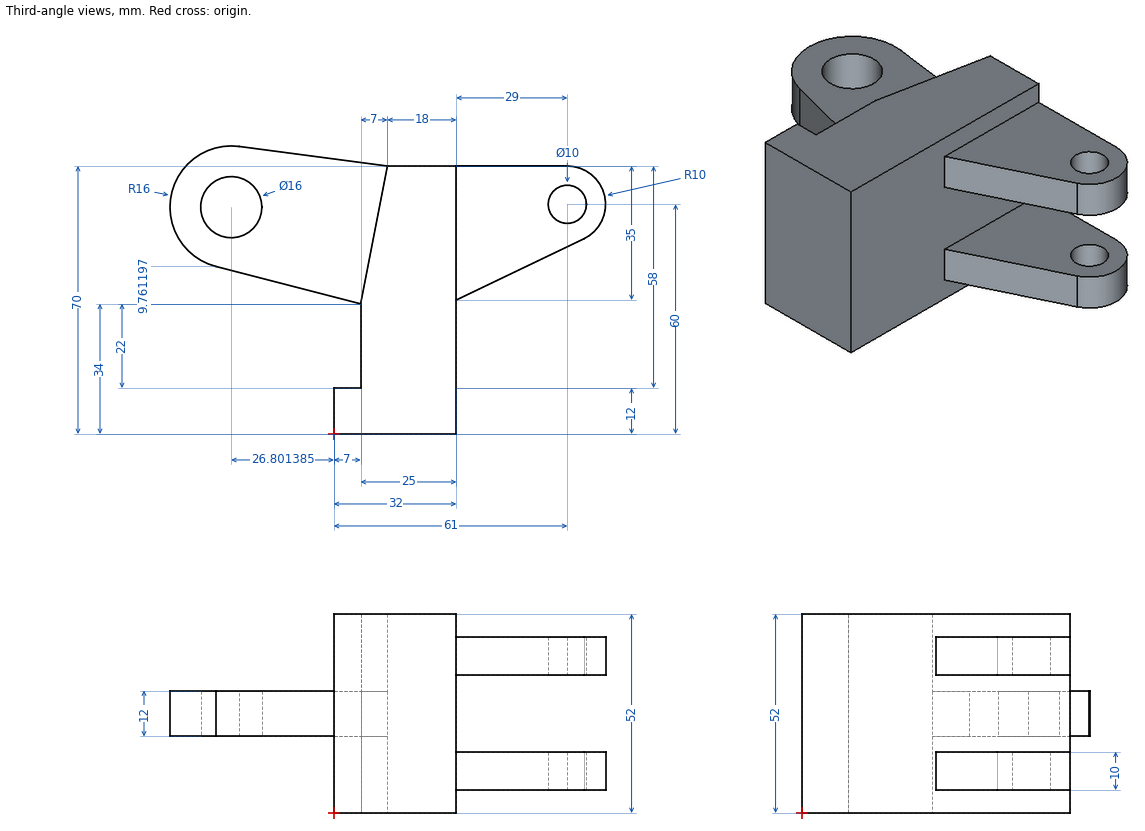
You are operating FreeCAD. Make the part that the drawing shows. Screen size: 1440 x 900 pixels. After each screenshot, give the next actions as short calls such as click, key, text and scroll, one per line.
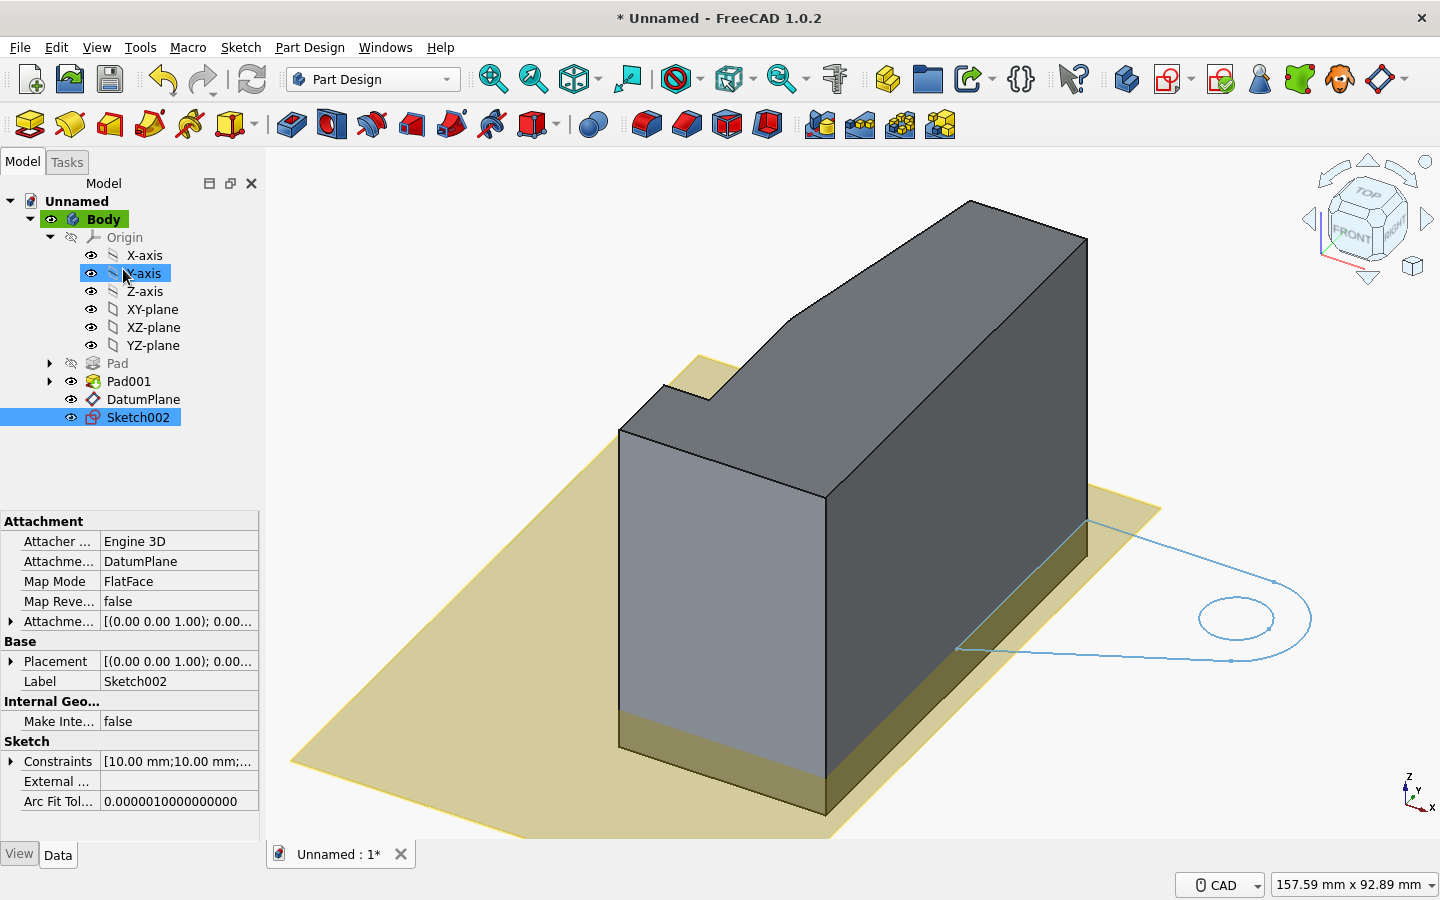
click(30, 124)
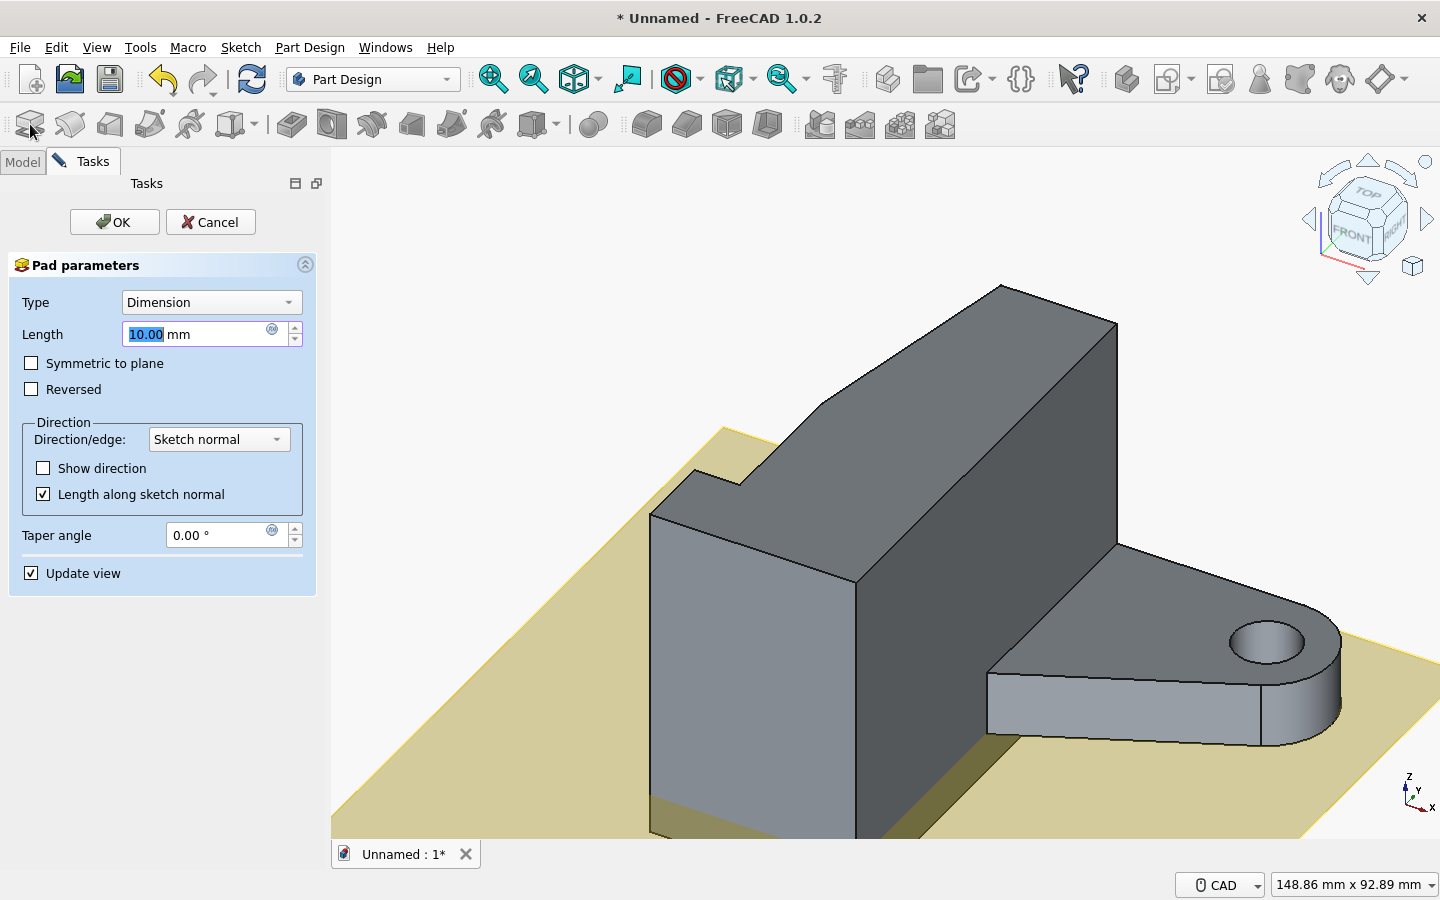
text(10)
key(Tab)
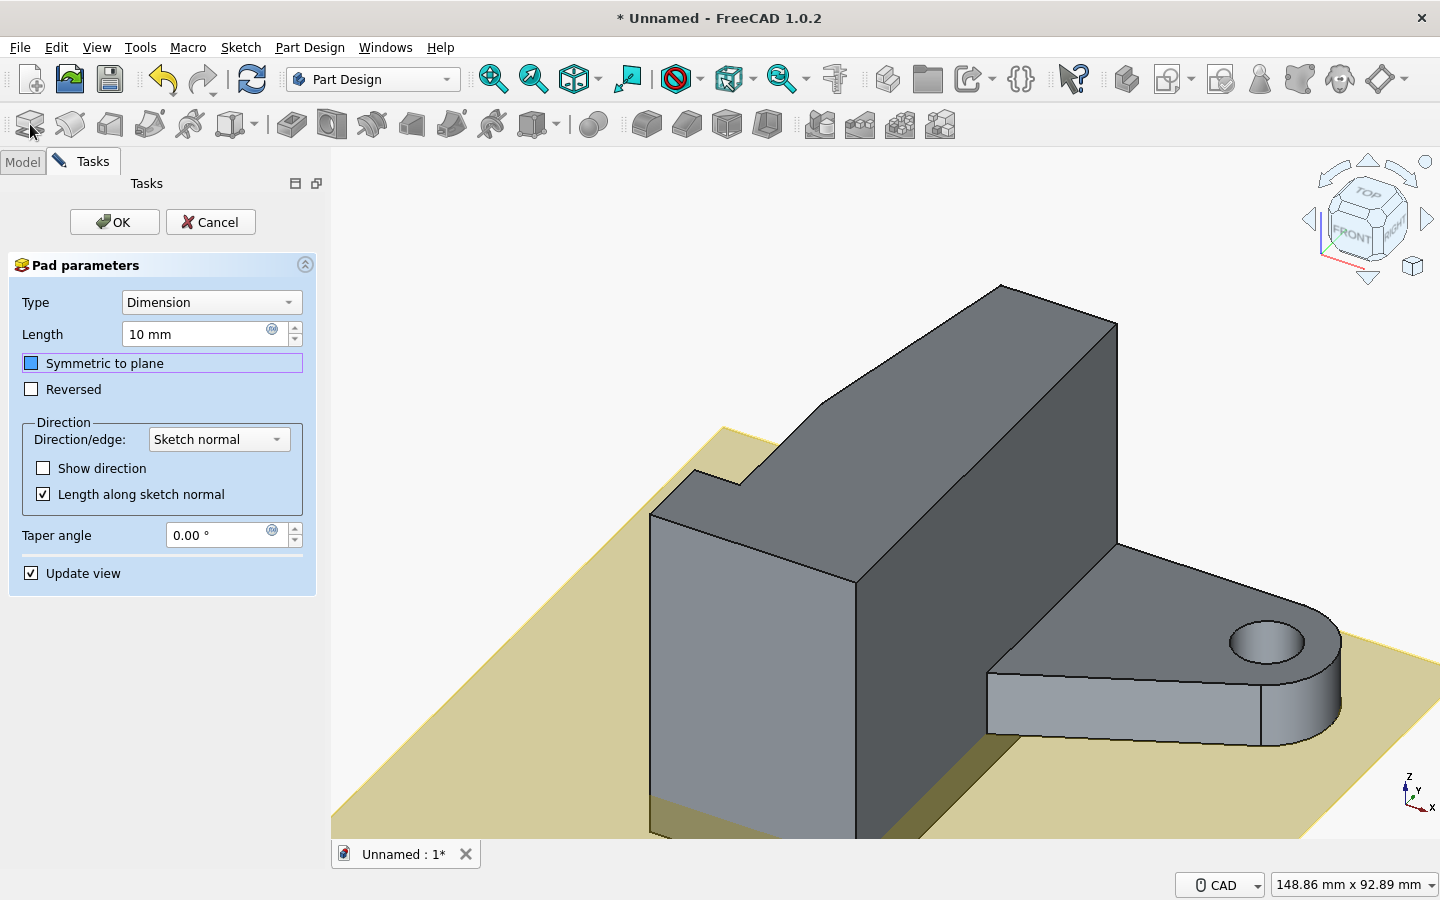
click(115, 222)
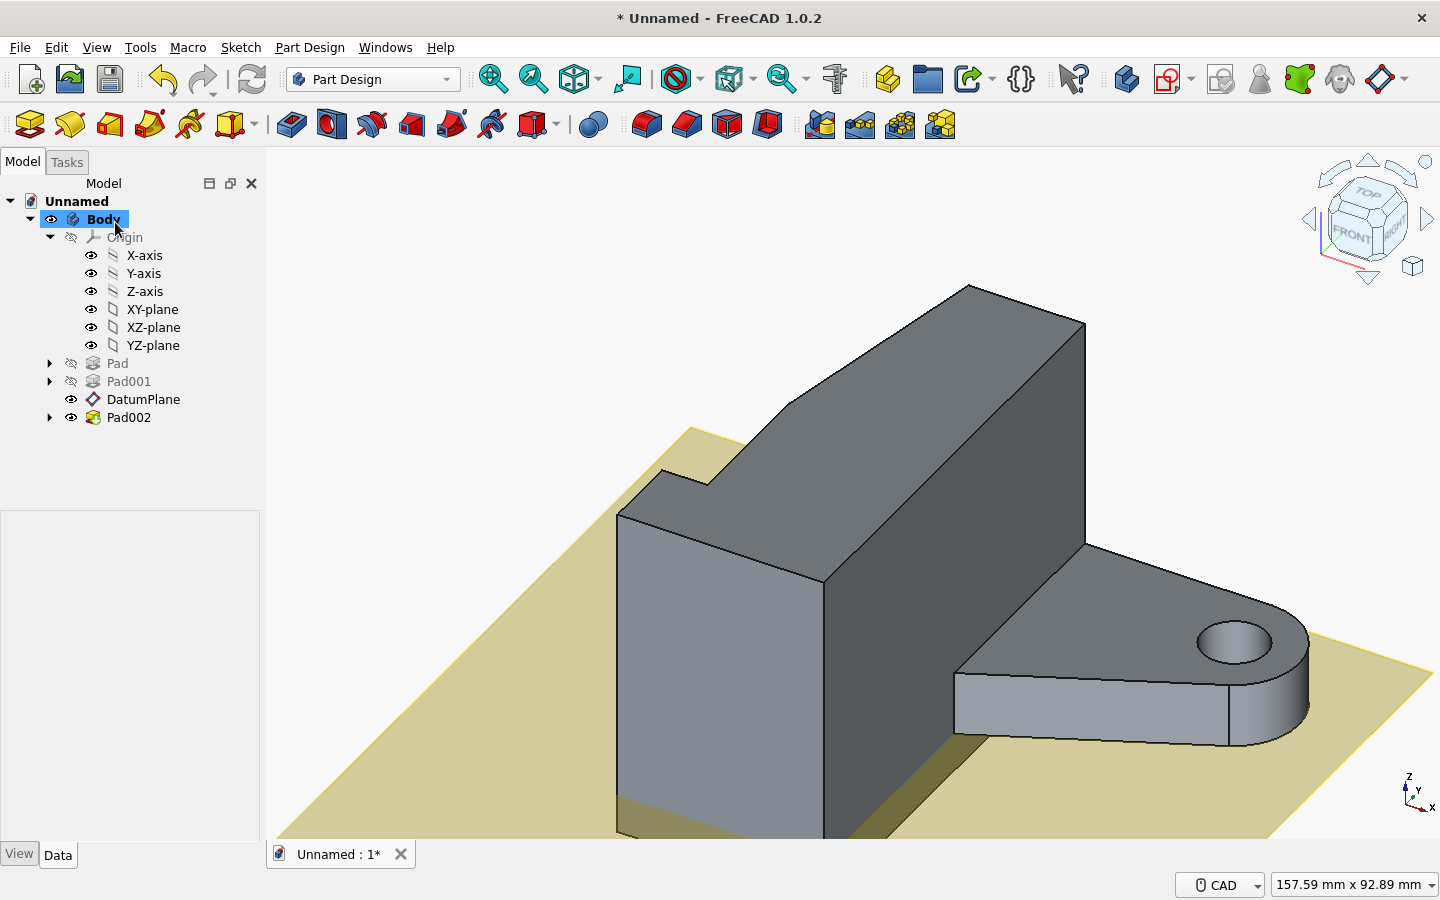
click(116, 399)
key(space)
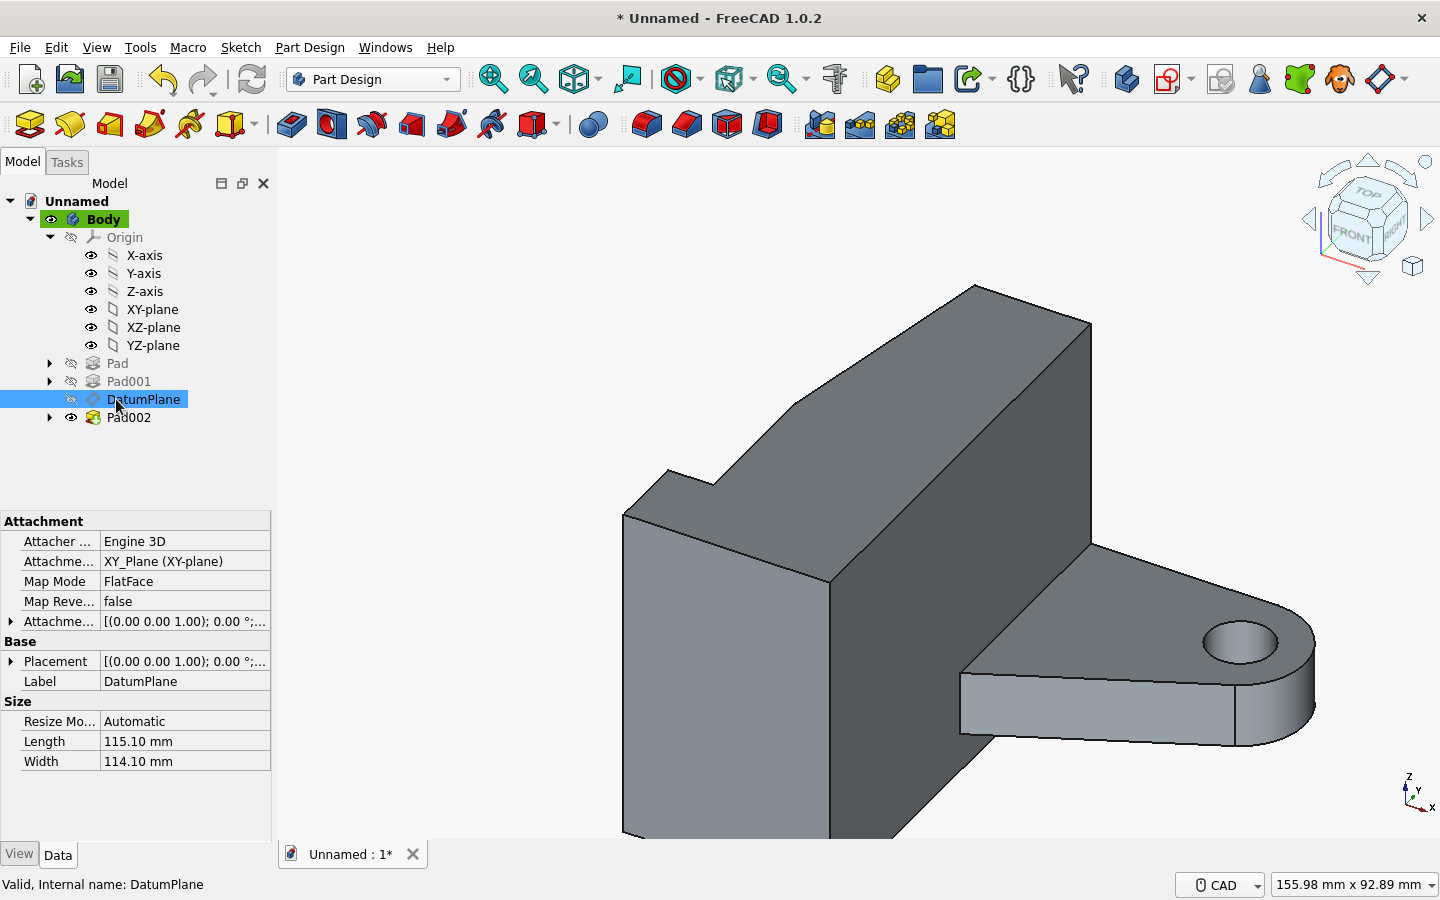
click(494, 80)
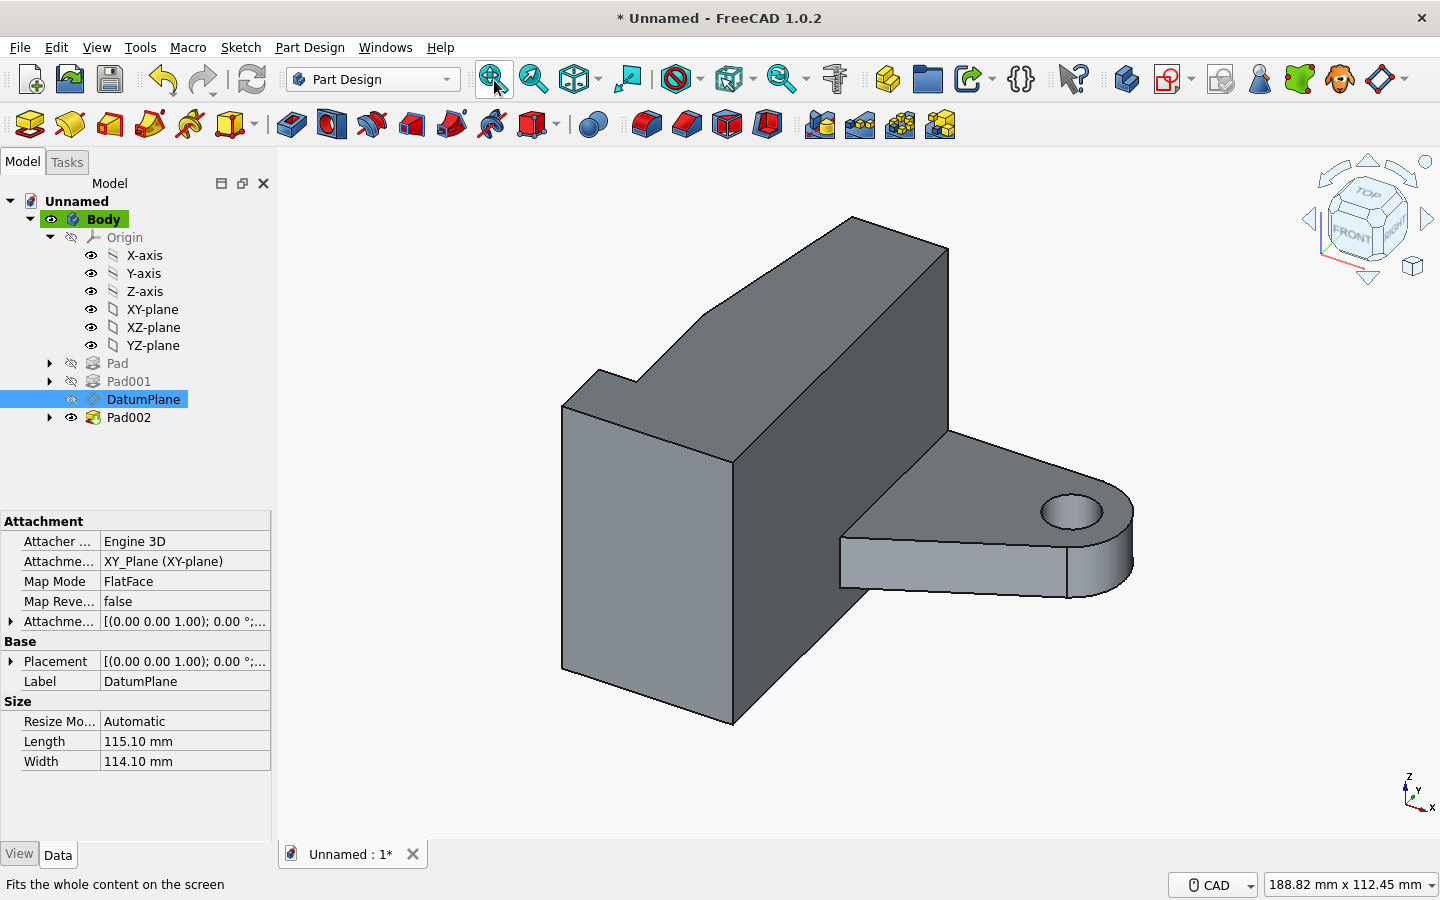
click(136, 309)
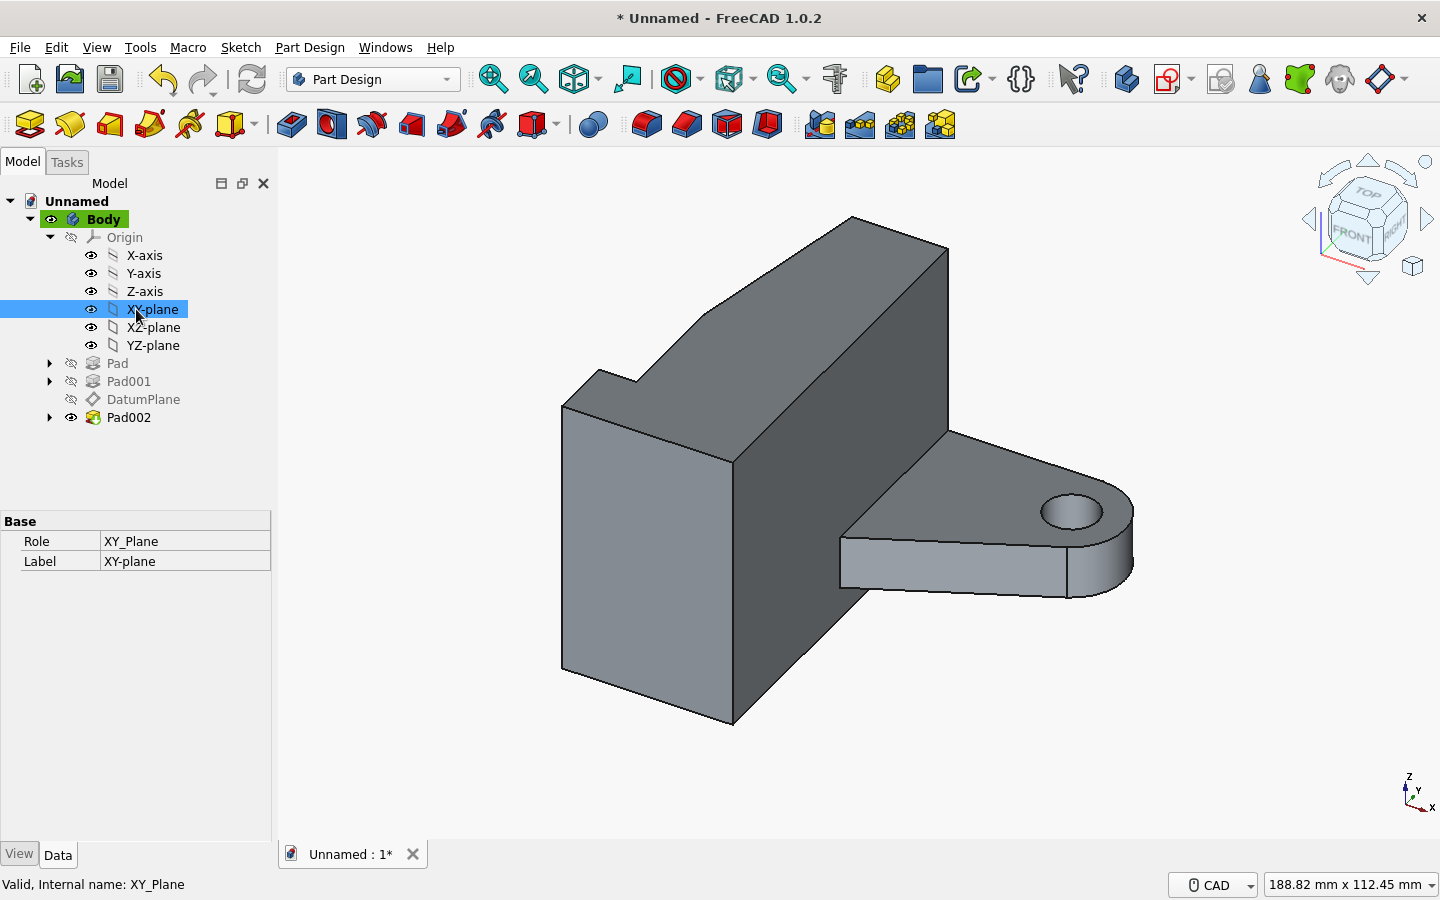
click(1380, 80)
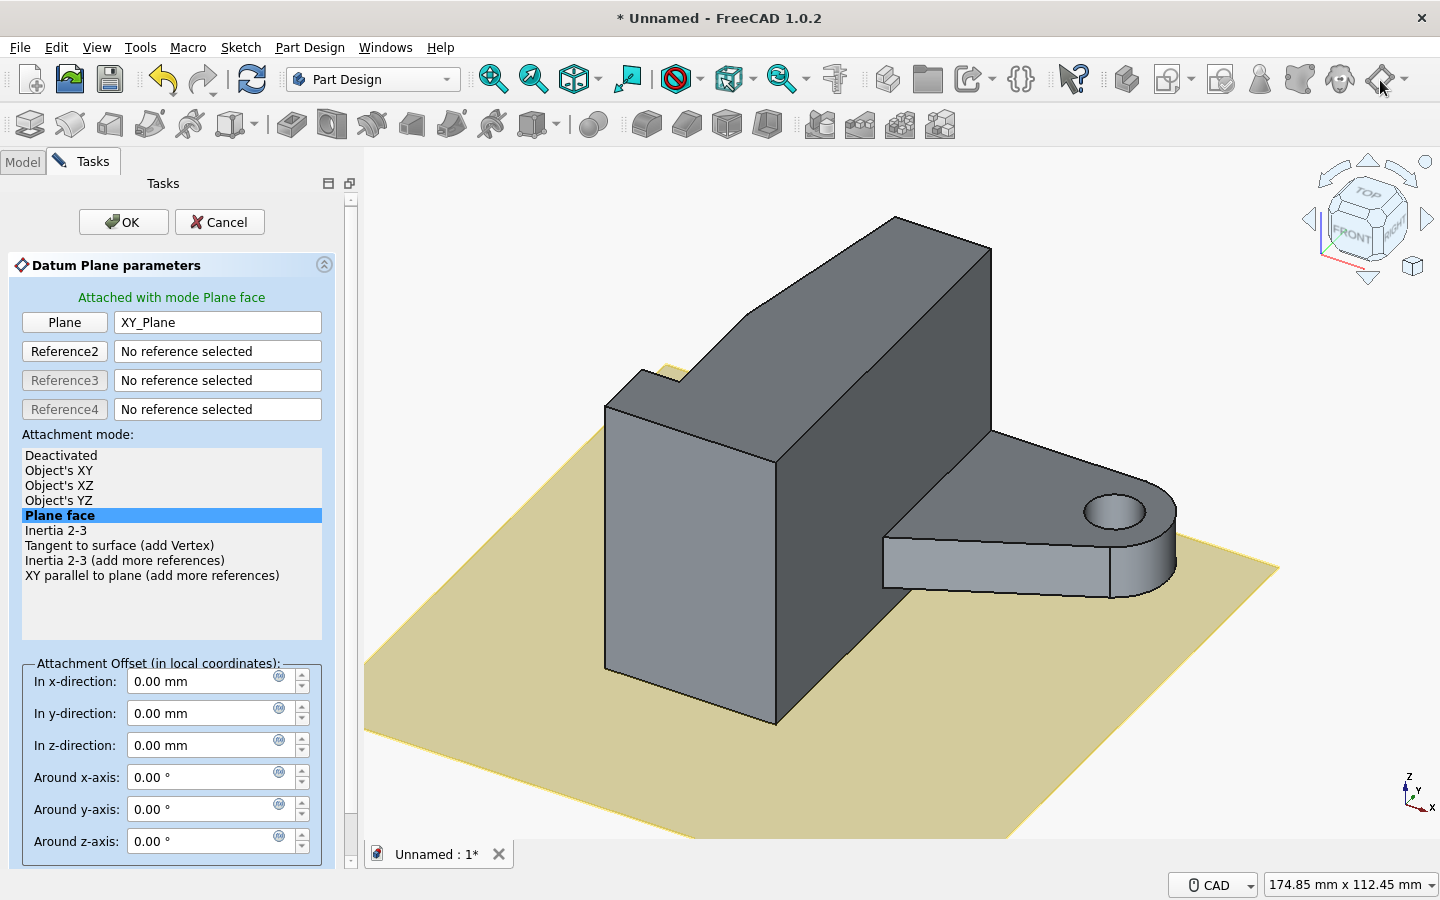
triple_click(210, 745)